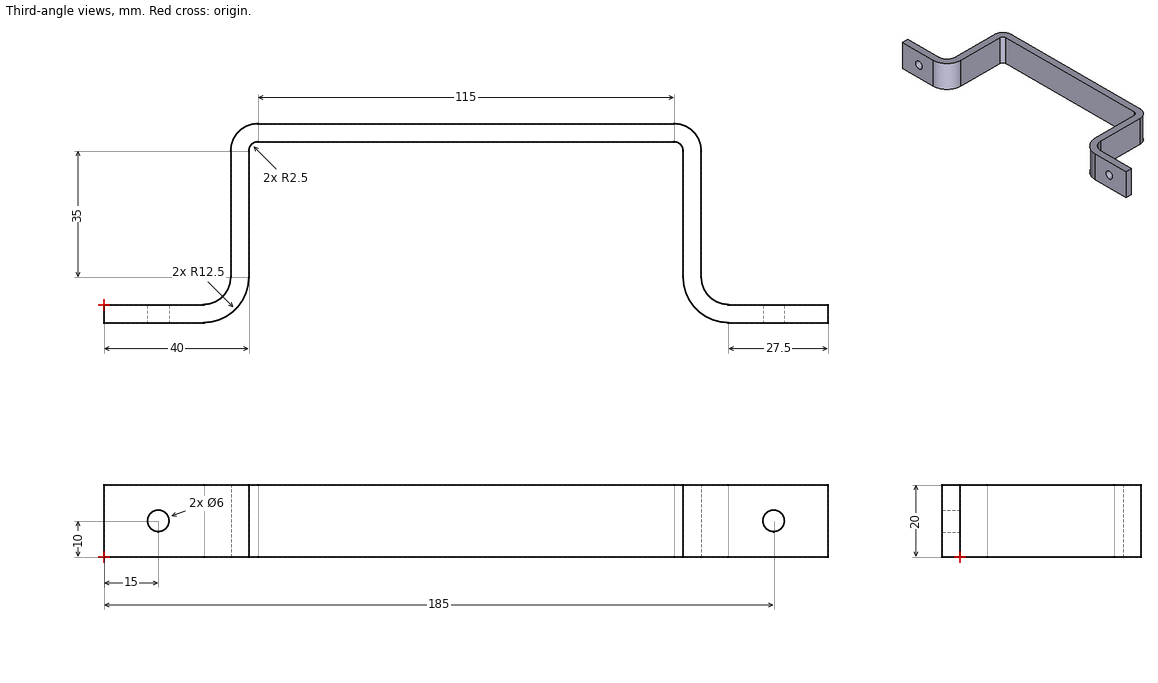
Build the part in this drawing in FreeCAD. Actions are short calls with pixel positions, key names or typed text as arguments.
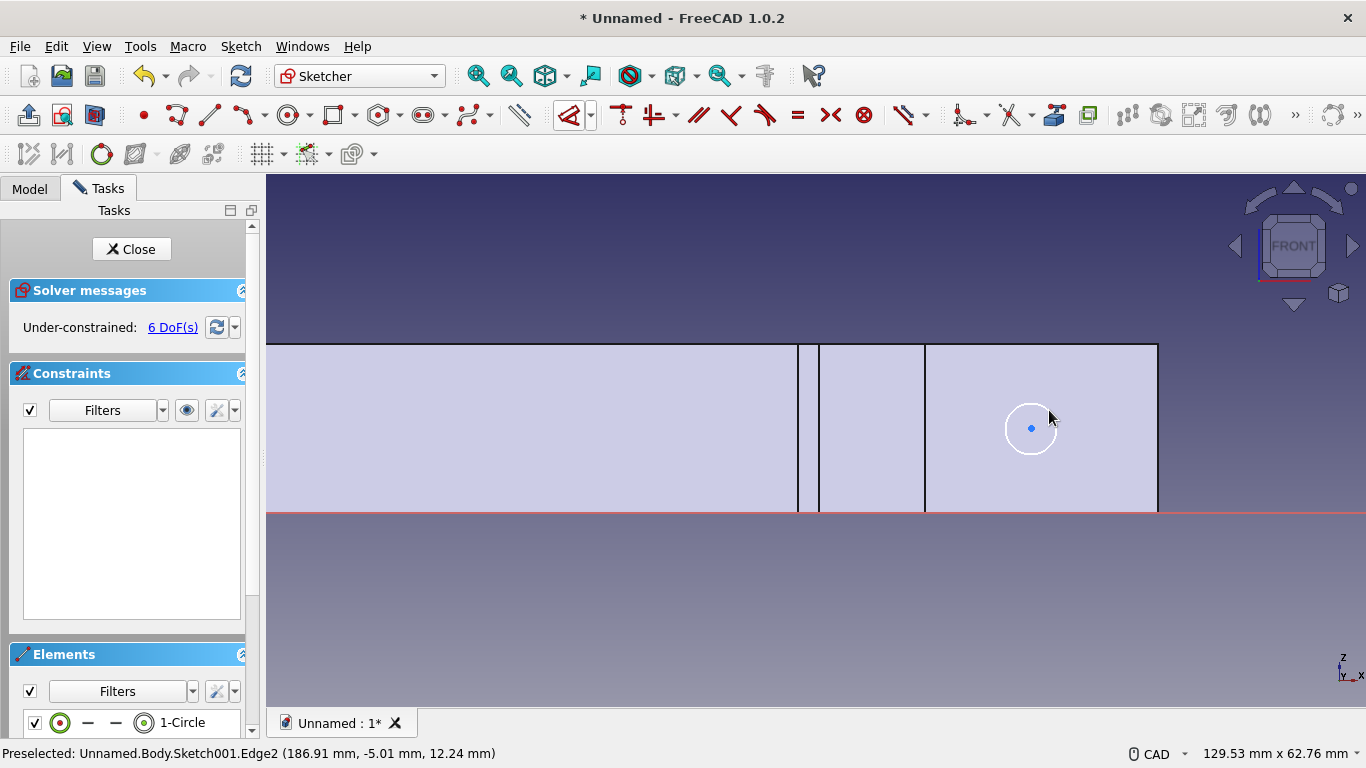
scroll(1032, 430, down, 5)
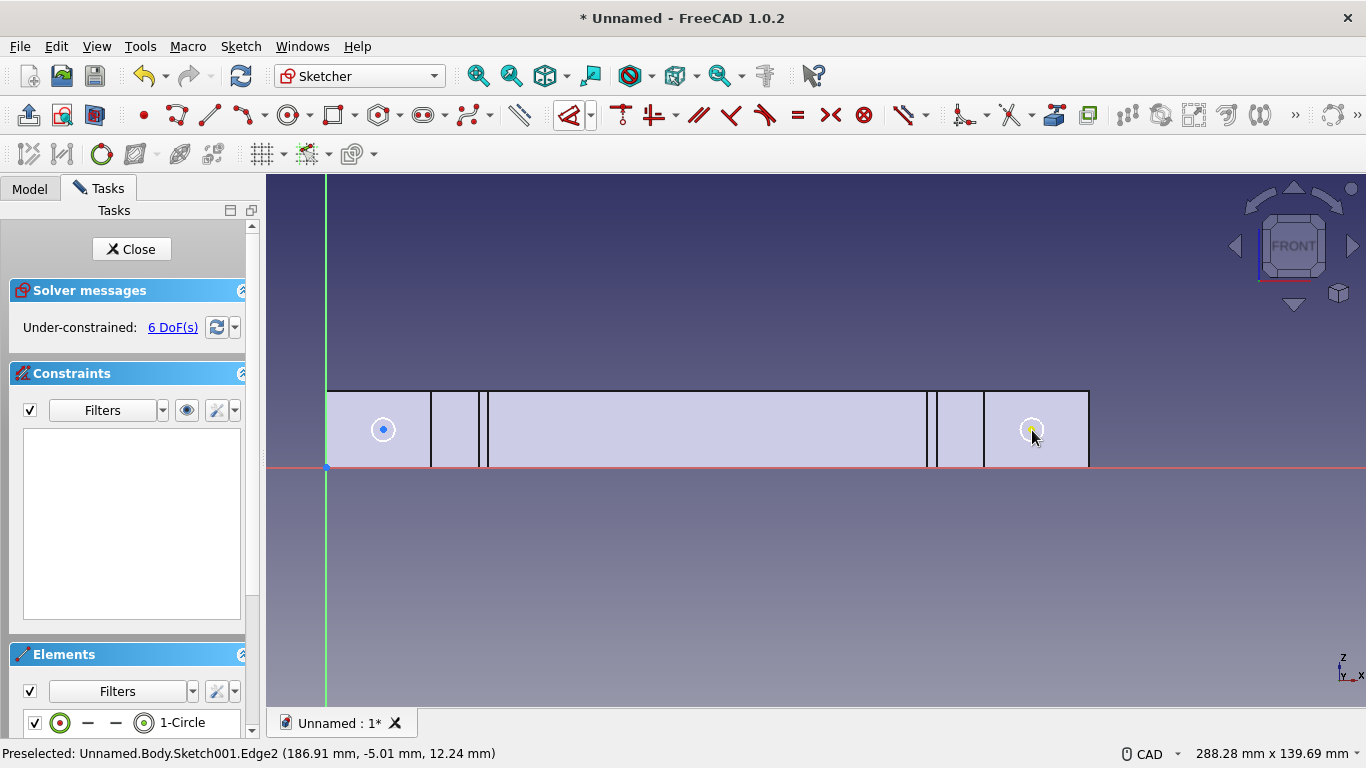
scroll(508, 423, up, 2)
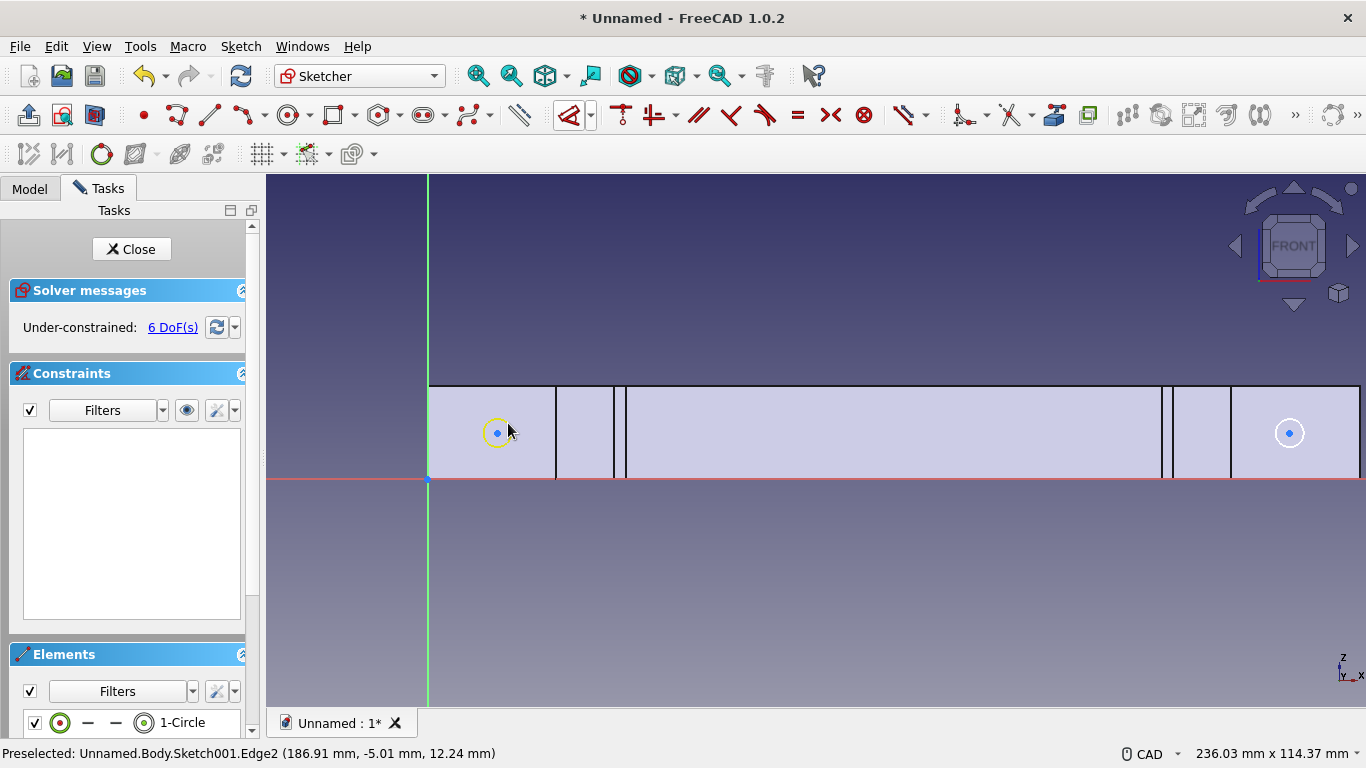
click(507, 423)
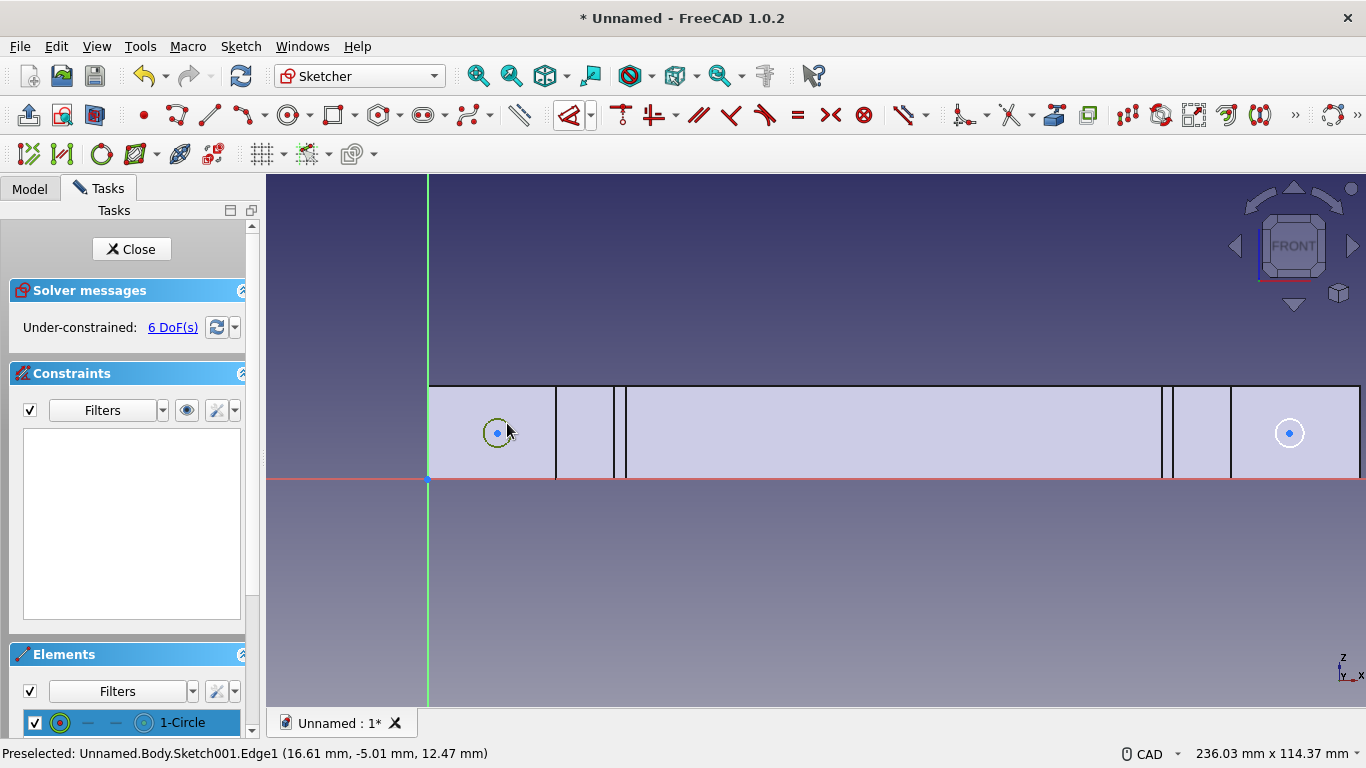
scroll(507, 423, down, 2)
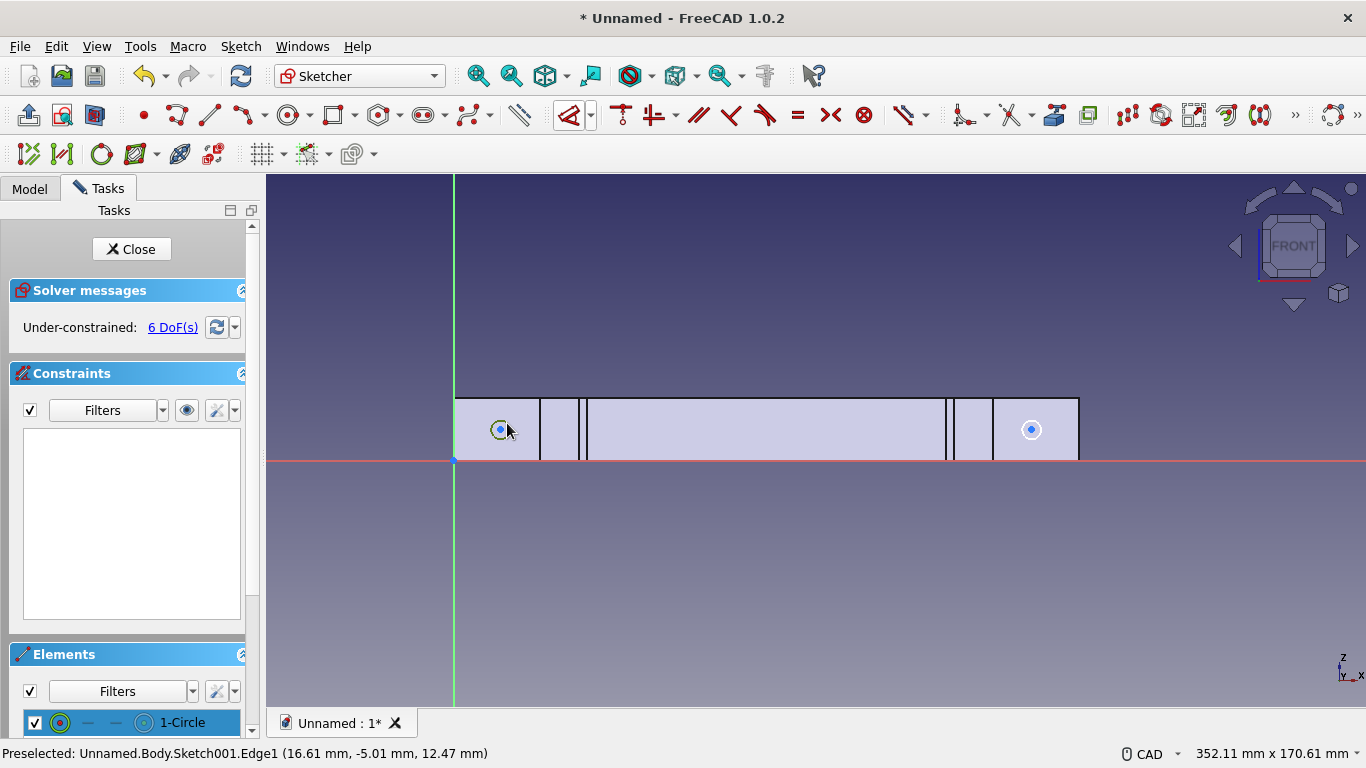
scroll(1038, 423, up, 2)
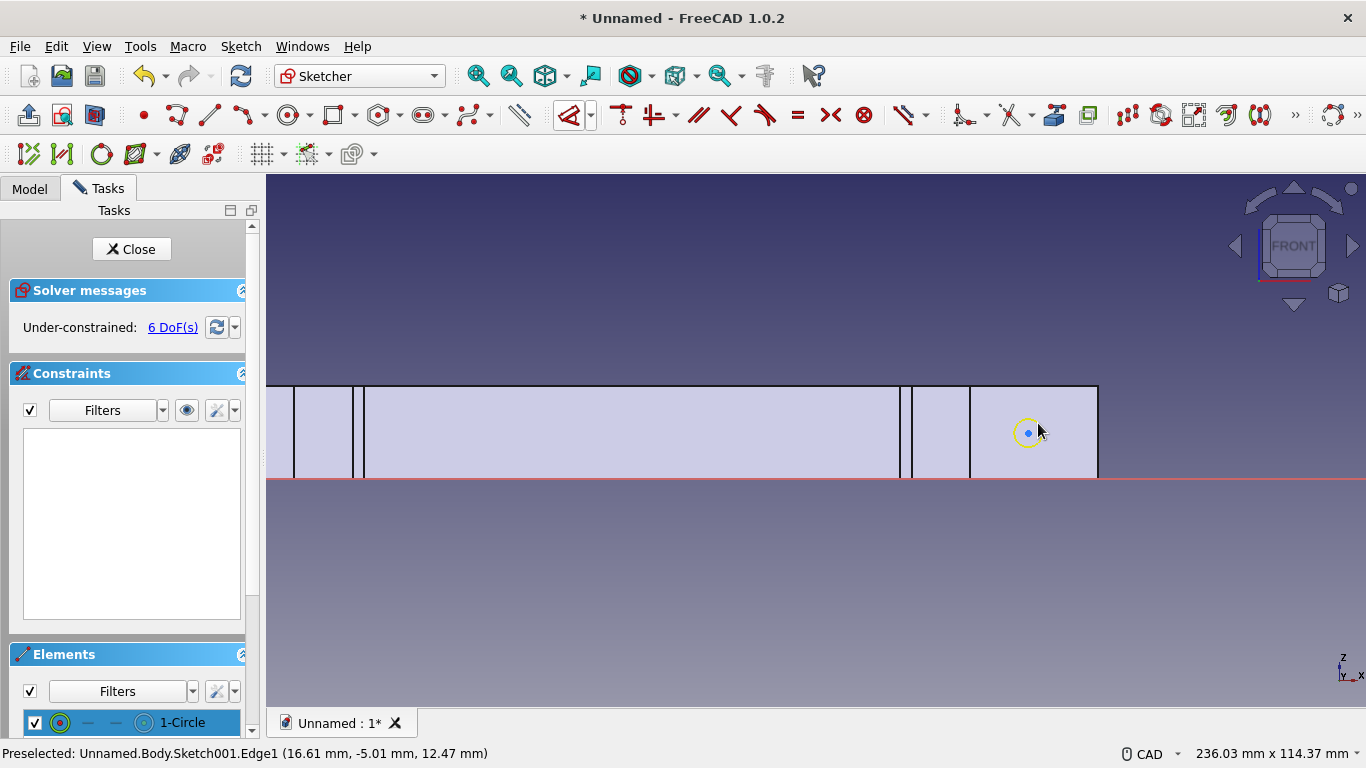
click(1038, 423)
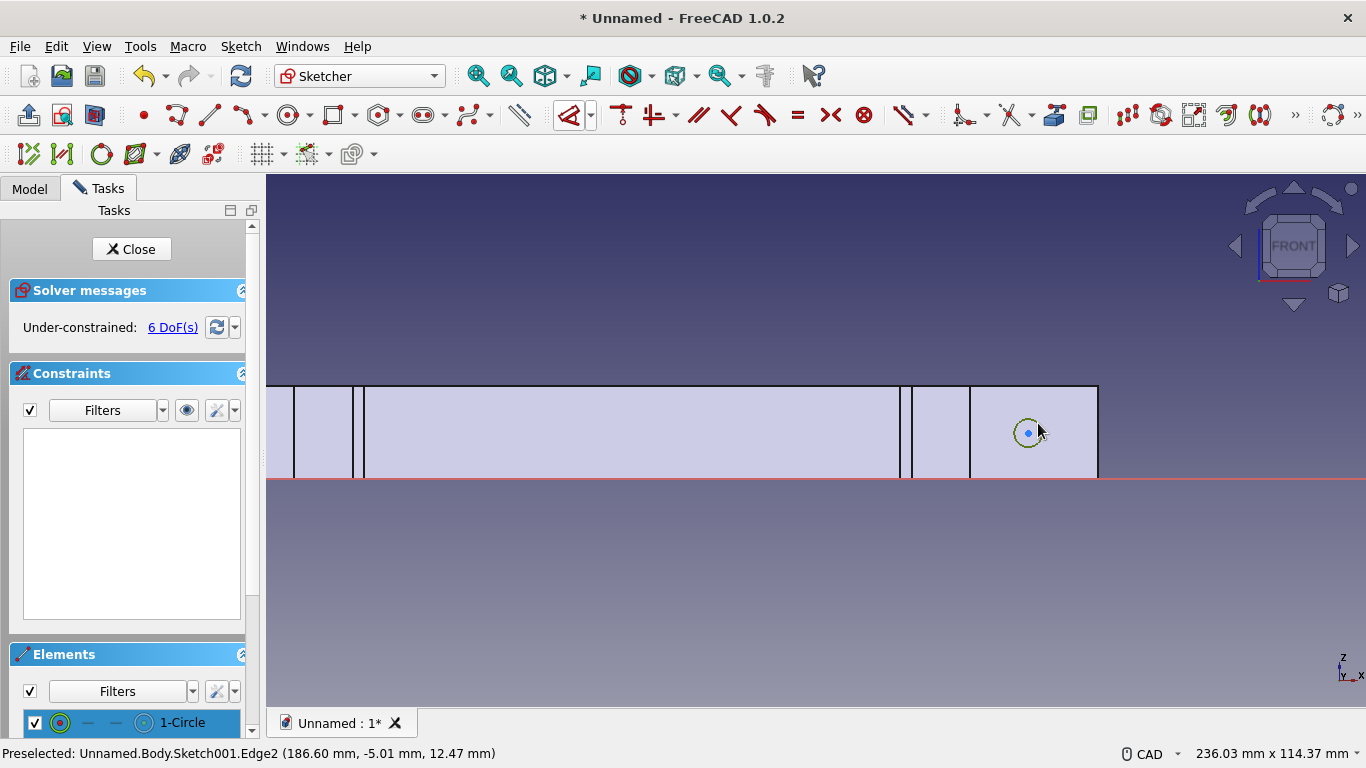
click(798, 116)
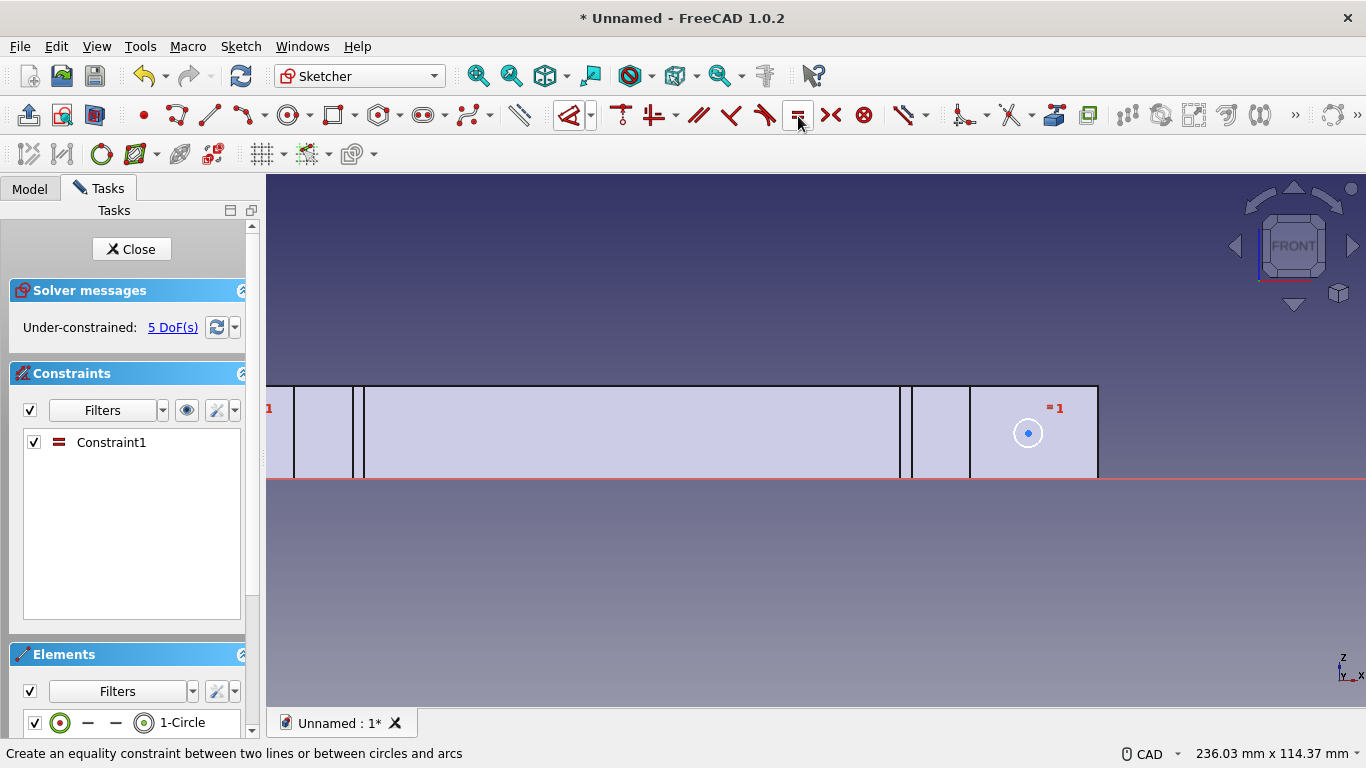
scroll(1039, 423, down, 2)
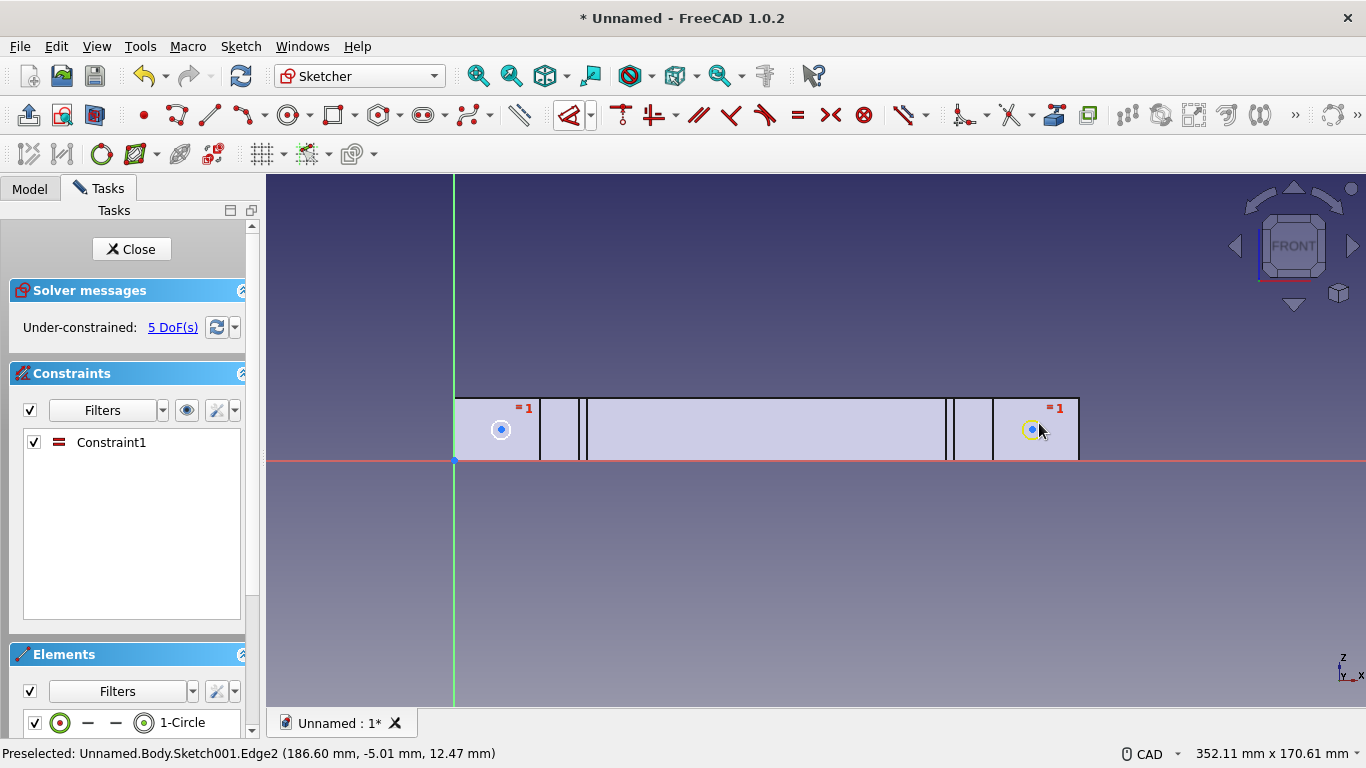
scroll(508, 423, up, 4)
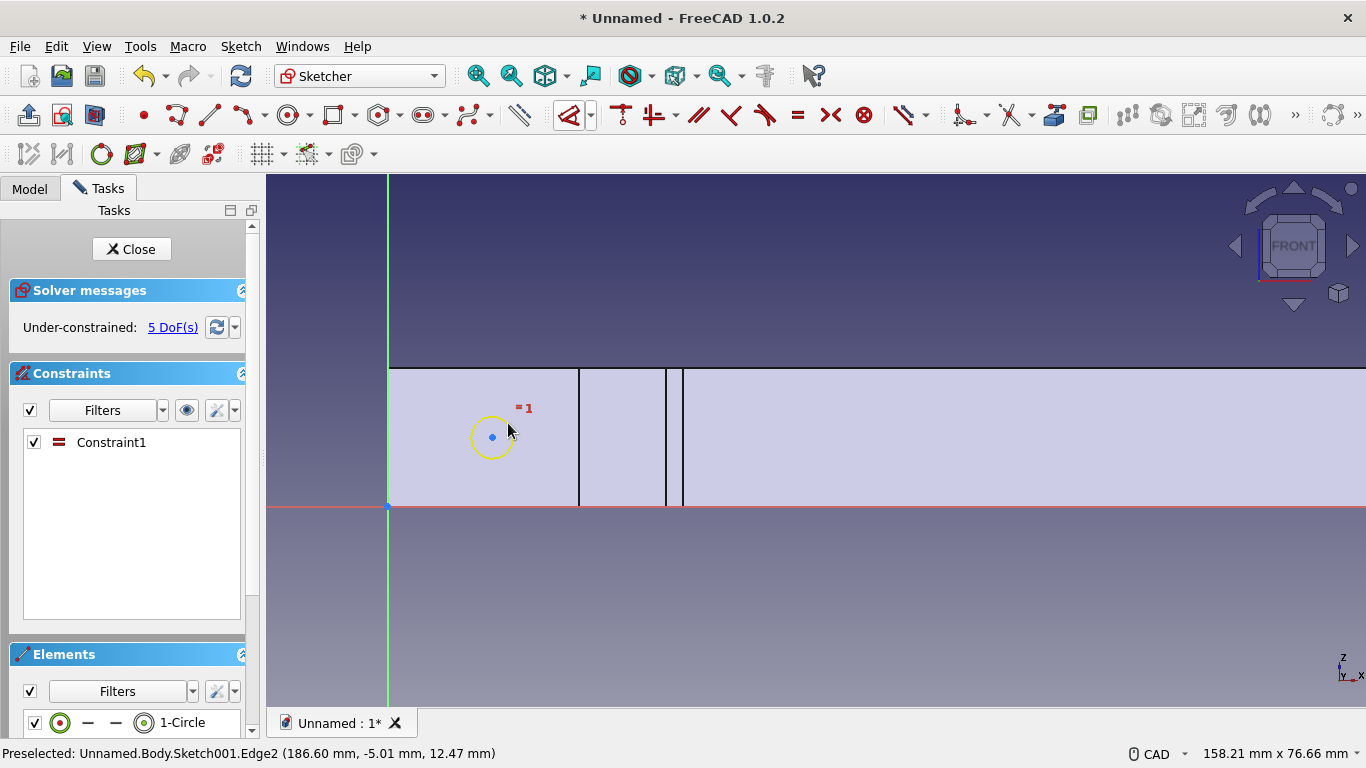
click(507, 423)